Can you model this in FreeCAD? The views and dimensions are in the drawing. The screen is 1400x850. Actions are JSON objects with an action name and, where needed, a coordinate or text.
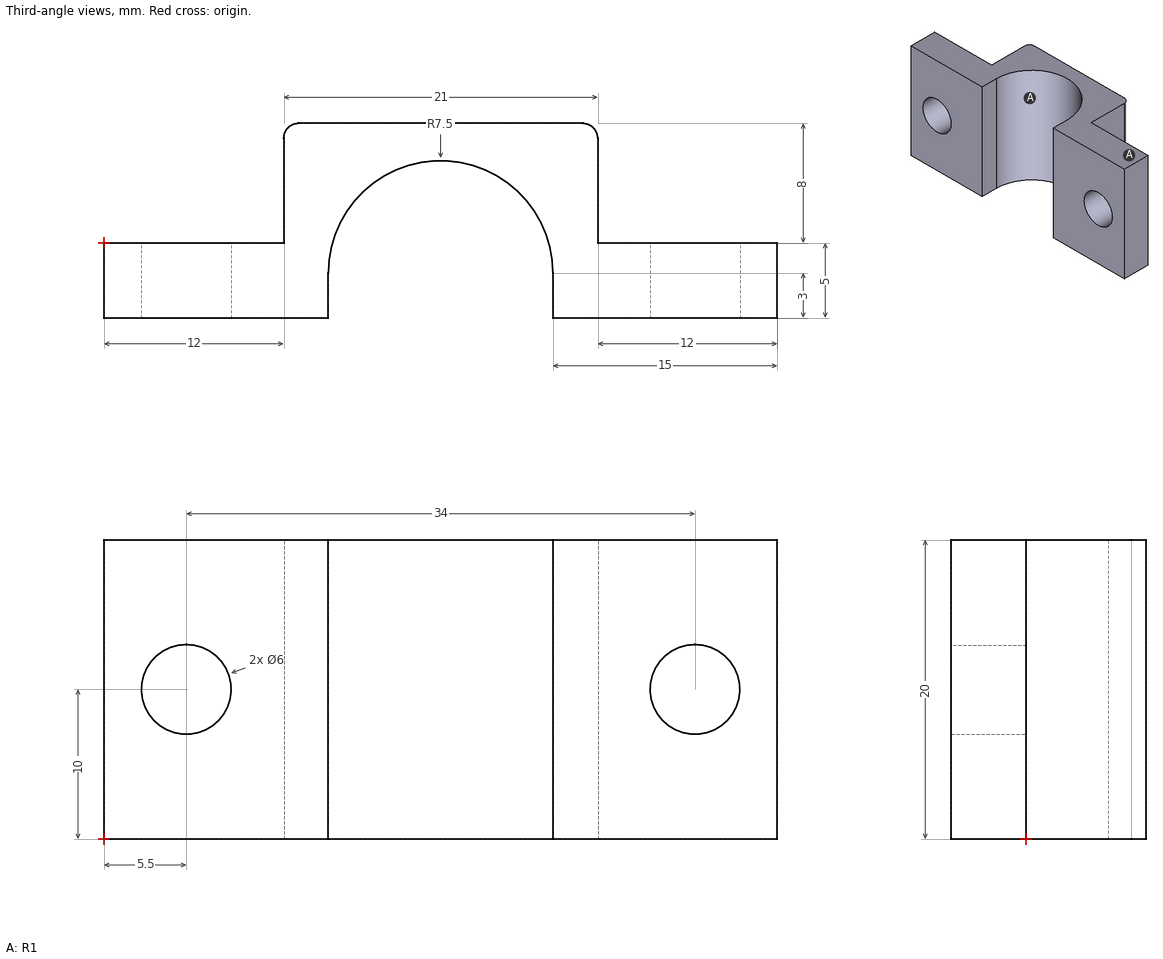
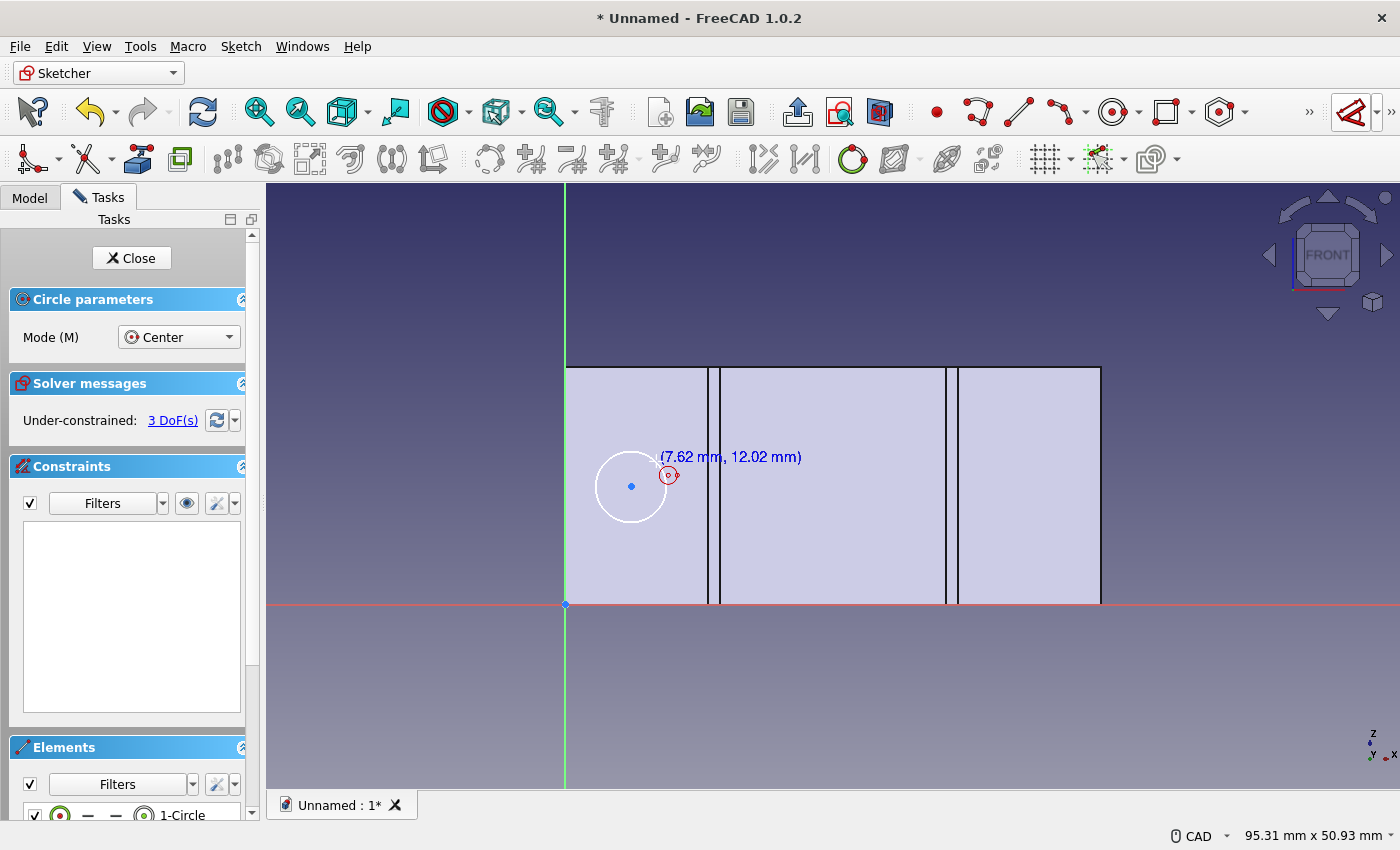
{"action": "left_click", "coordinate": [1035, 486]}
{"action": "left_click", "coordinate": [1061, 461]}
{"action": "key", "text": "Escape"}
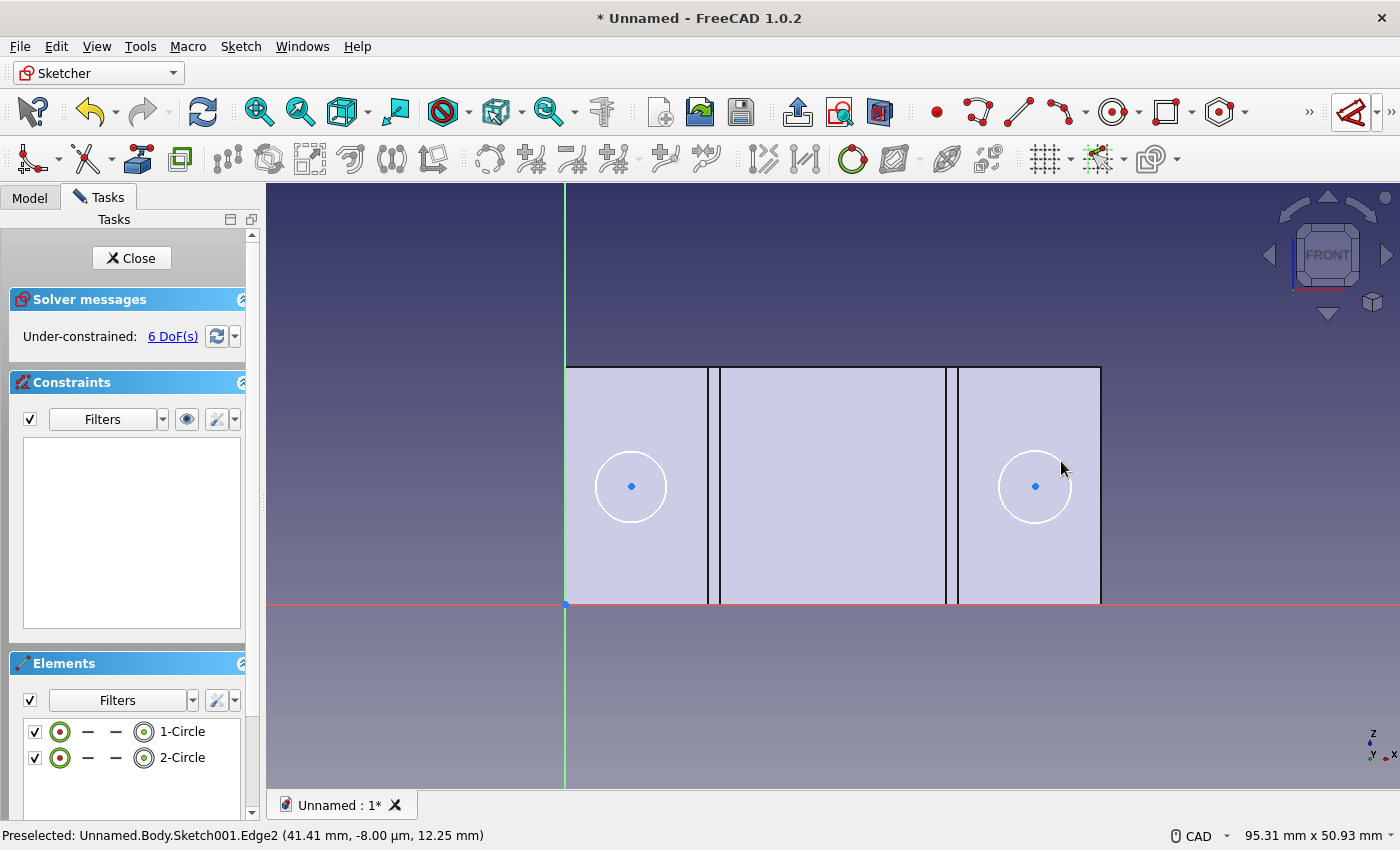
{"action": "left_click", "coordinate": [656, 462]}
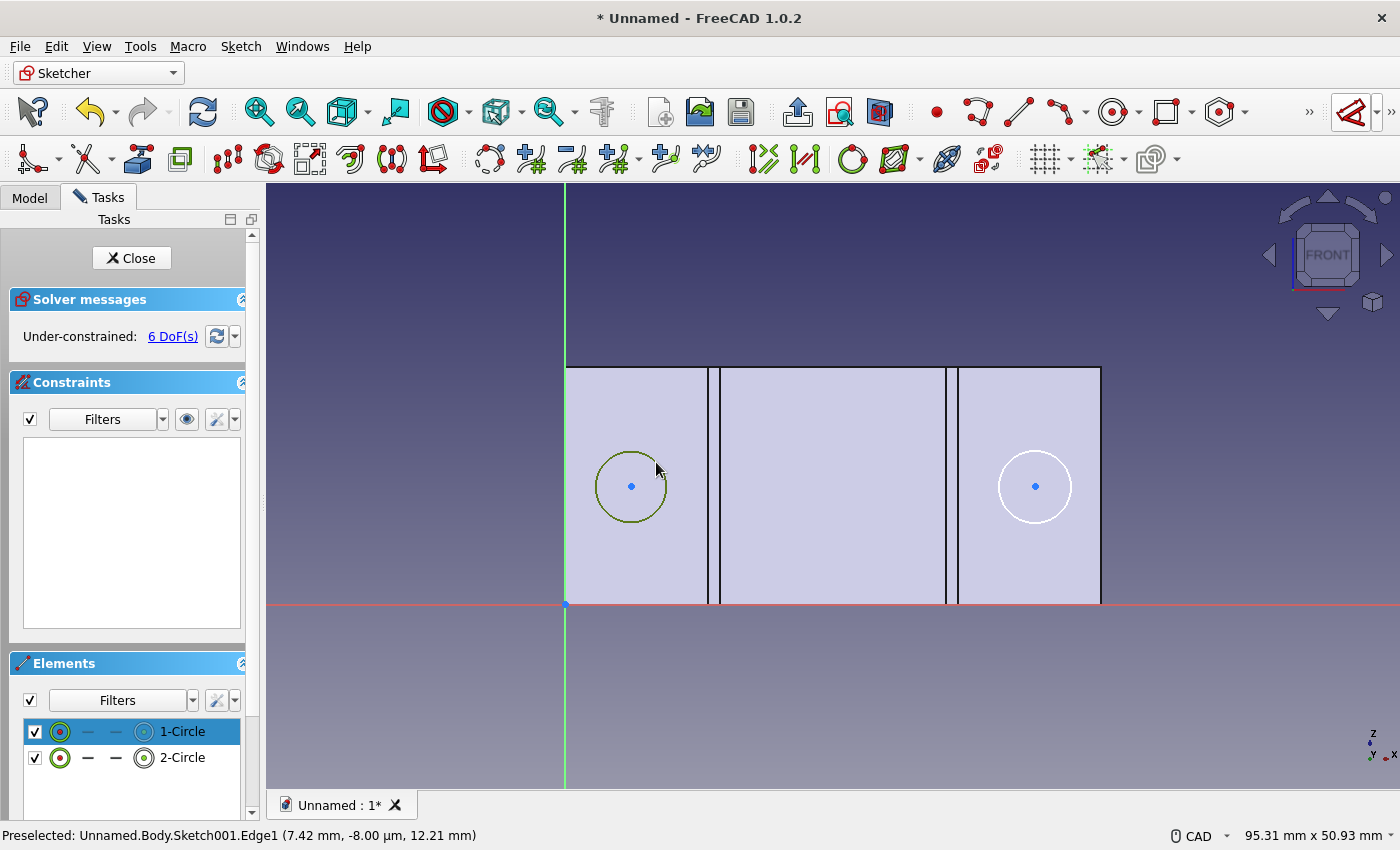
{"action": "left_click", "coordinate": [1060, 461]}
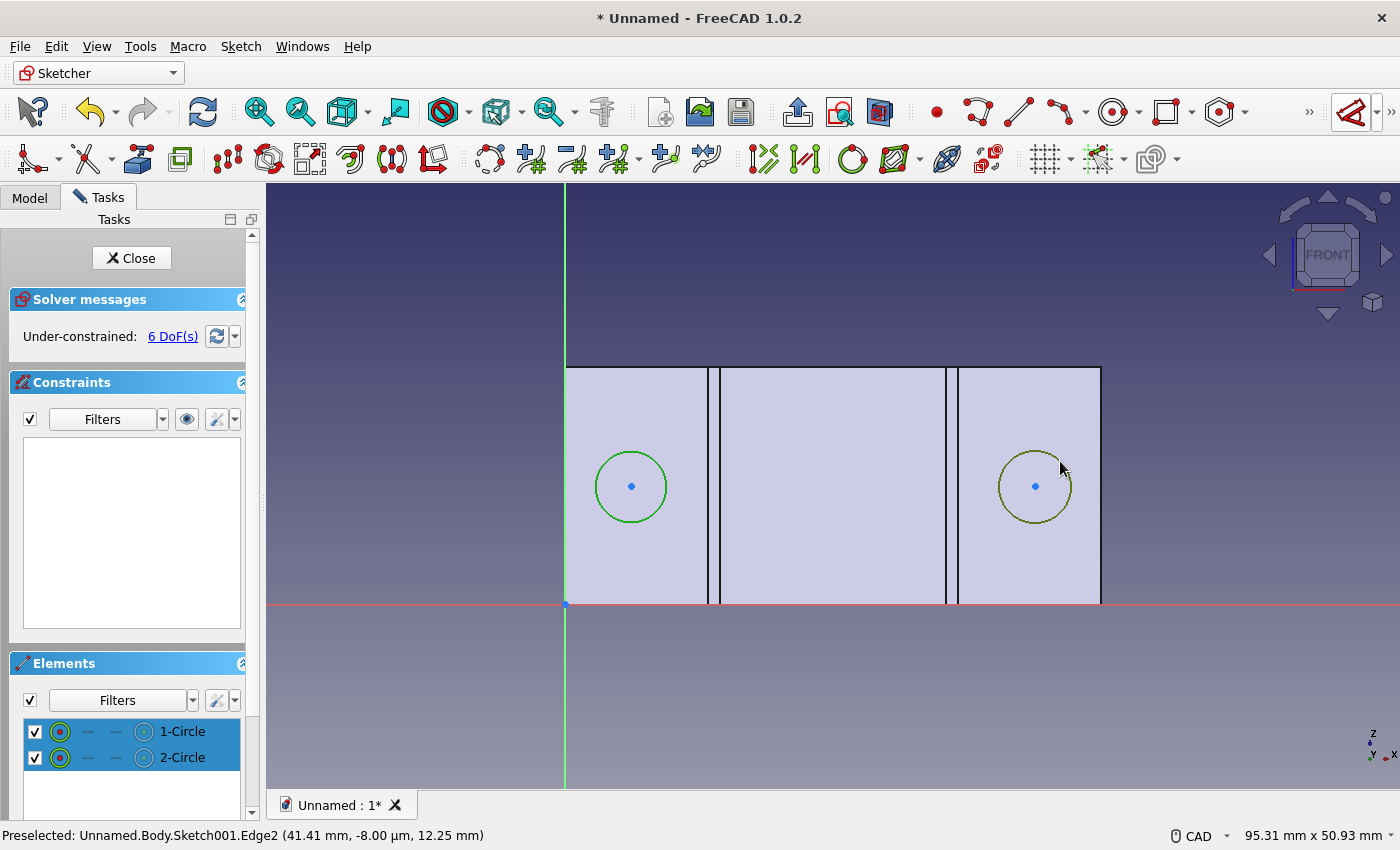
{"action": "key", "text": "e"}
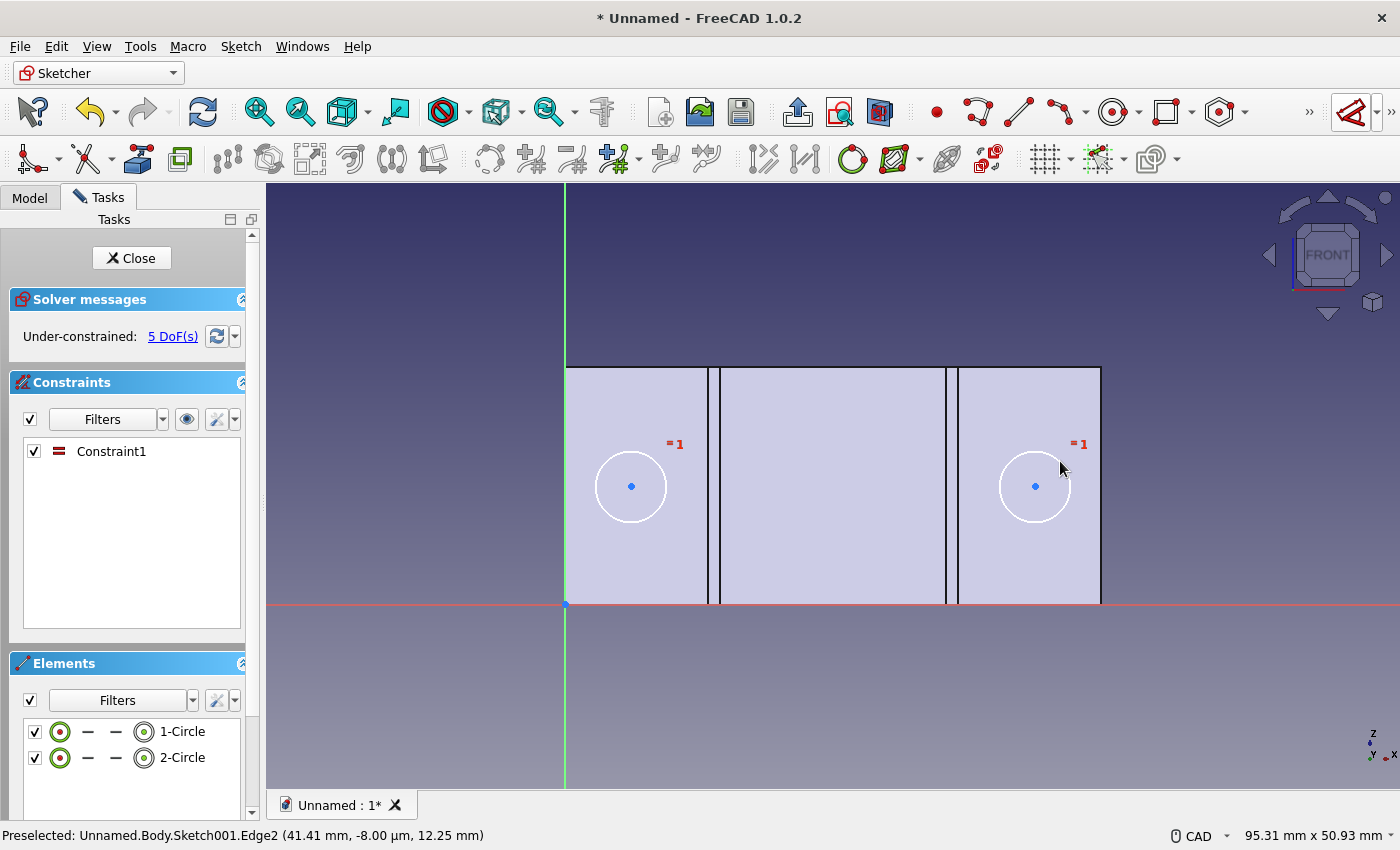
{"action": "left_click", "coordinate": [656, 462]}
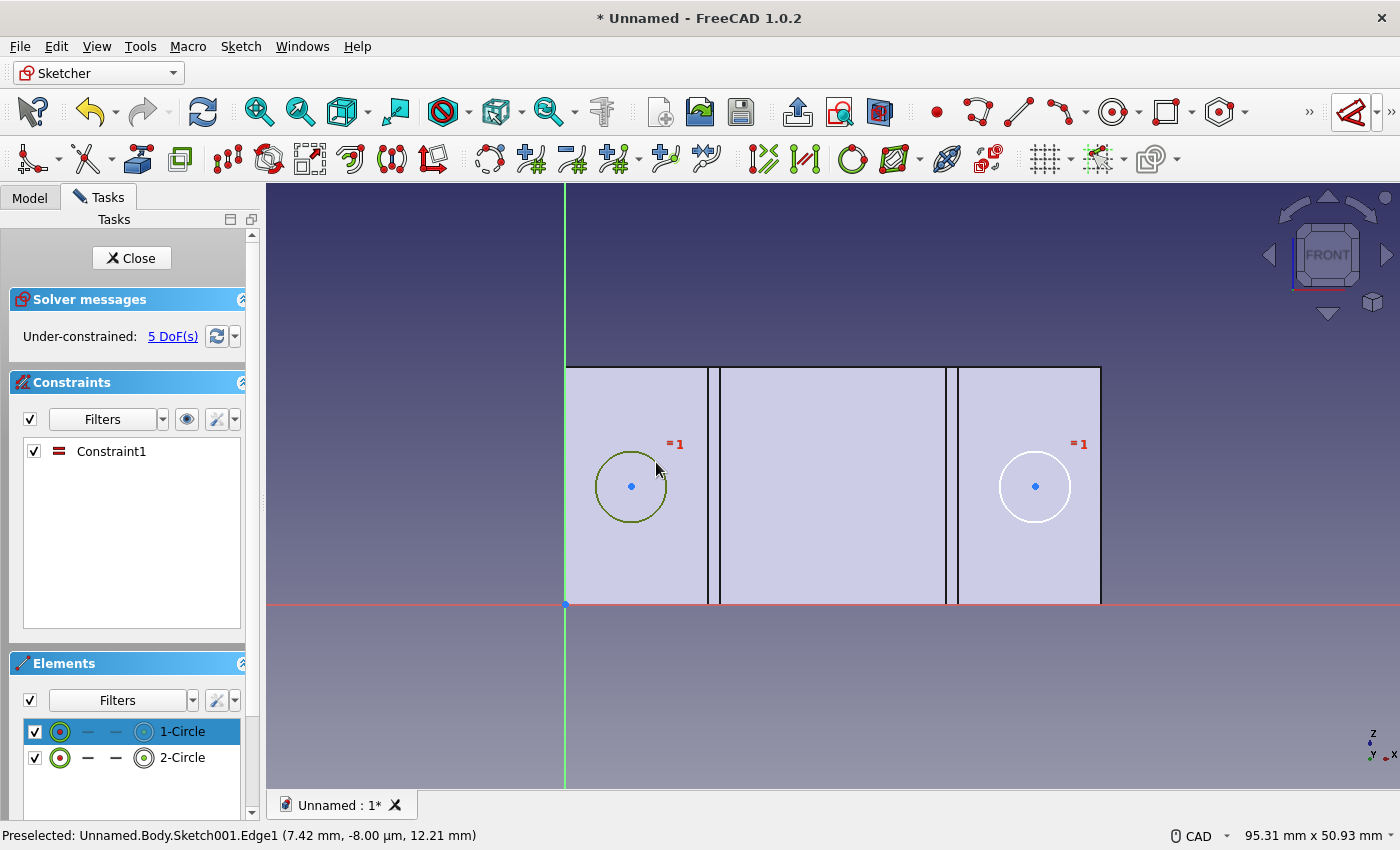
{"action": "left_click", "coordinate": [1376, 112]}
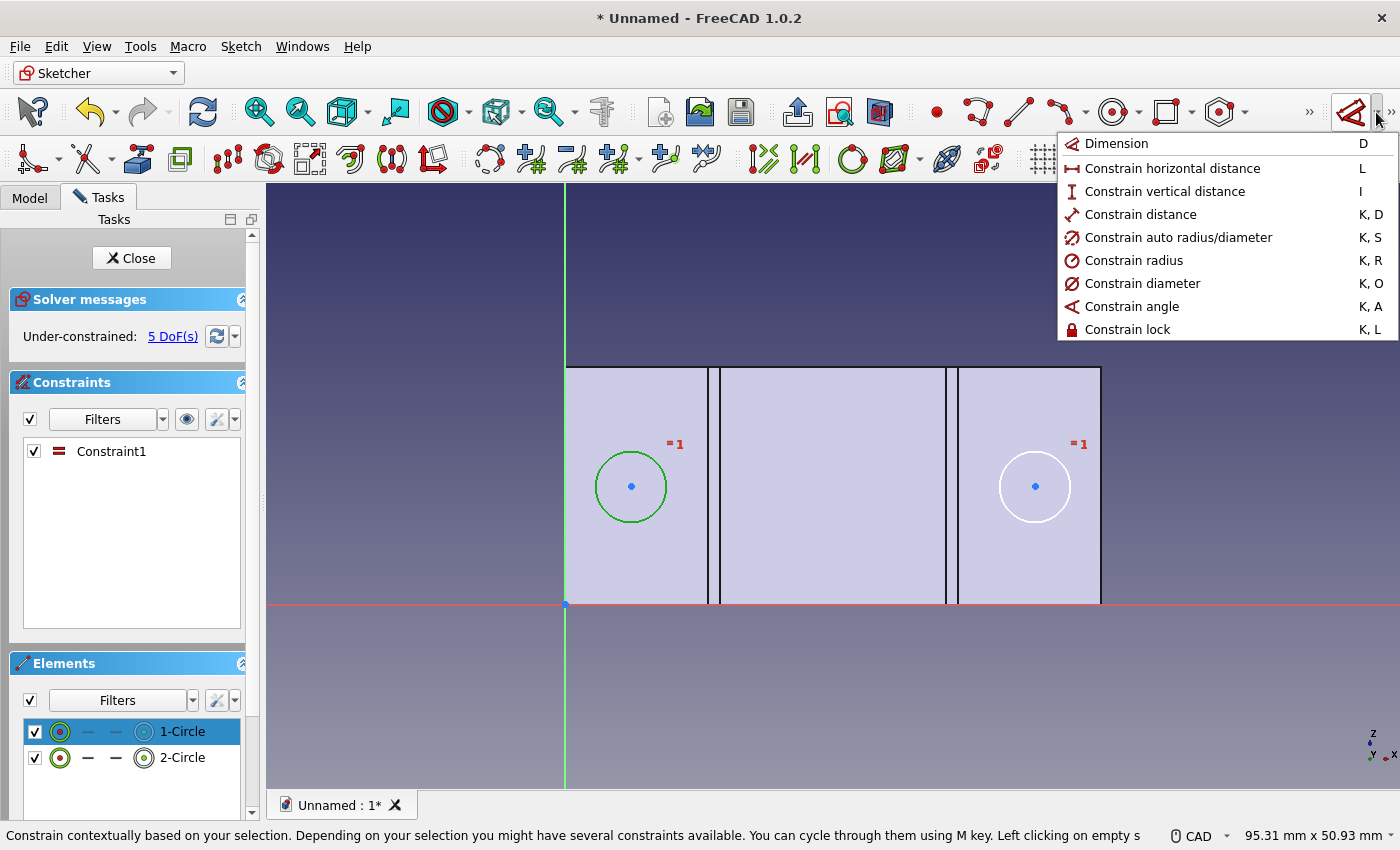
{"action": "left_click", "coordinate": [1228, 284]}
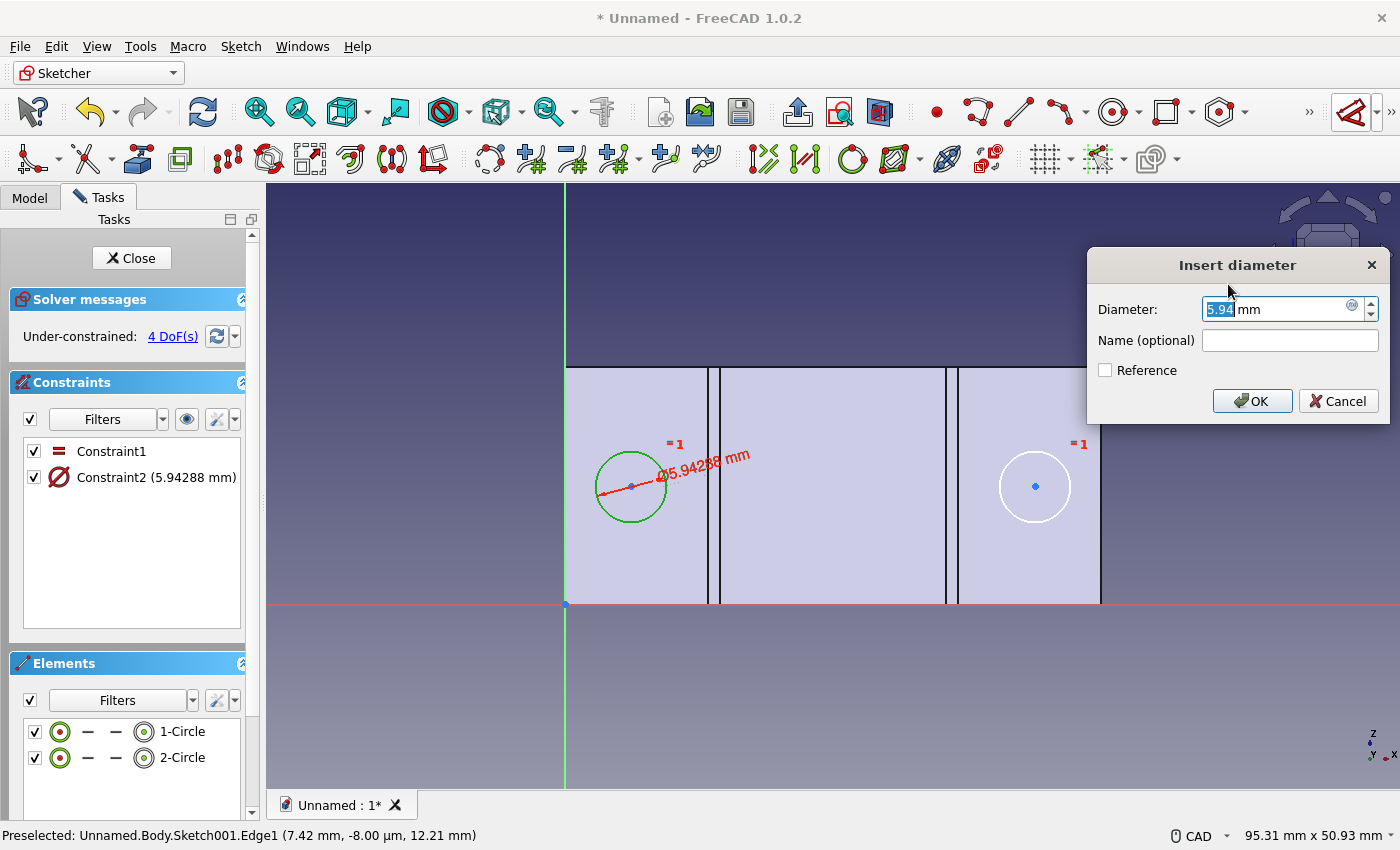
{"action": "type", "text": "6"}
{"action": "key", "text": "Return"}